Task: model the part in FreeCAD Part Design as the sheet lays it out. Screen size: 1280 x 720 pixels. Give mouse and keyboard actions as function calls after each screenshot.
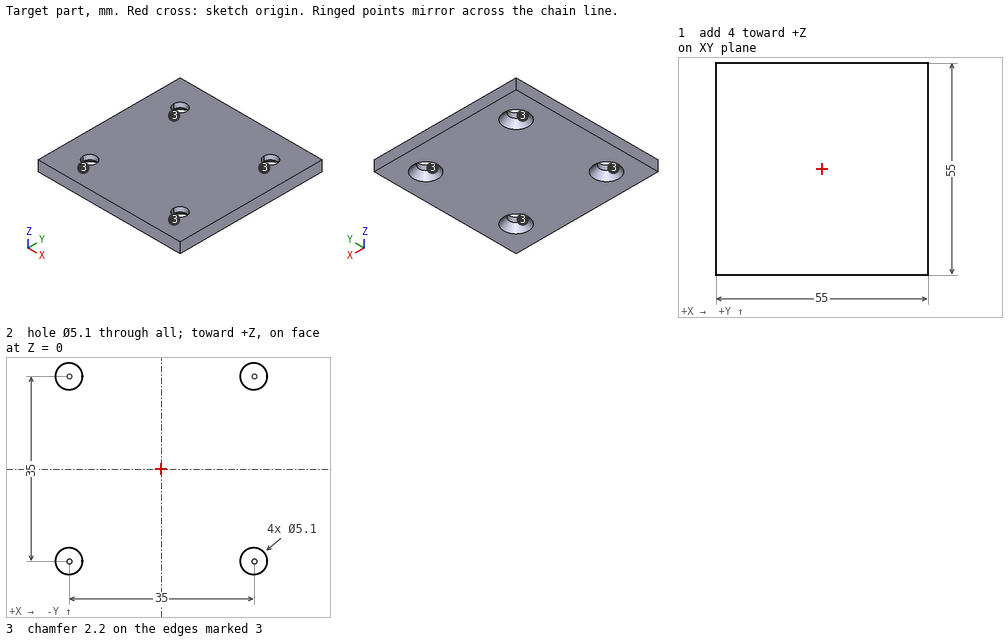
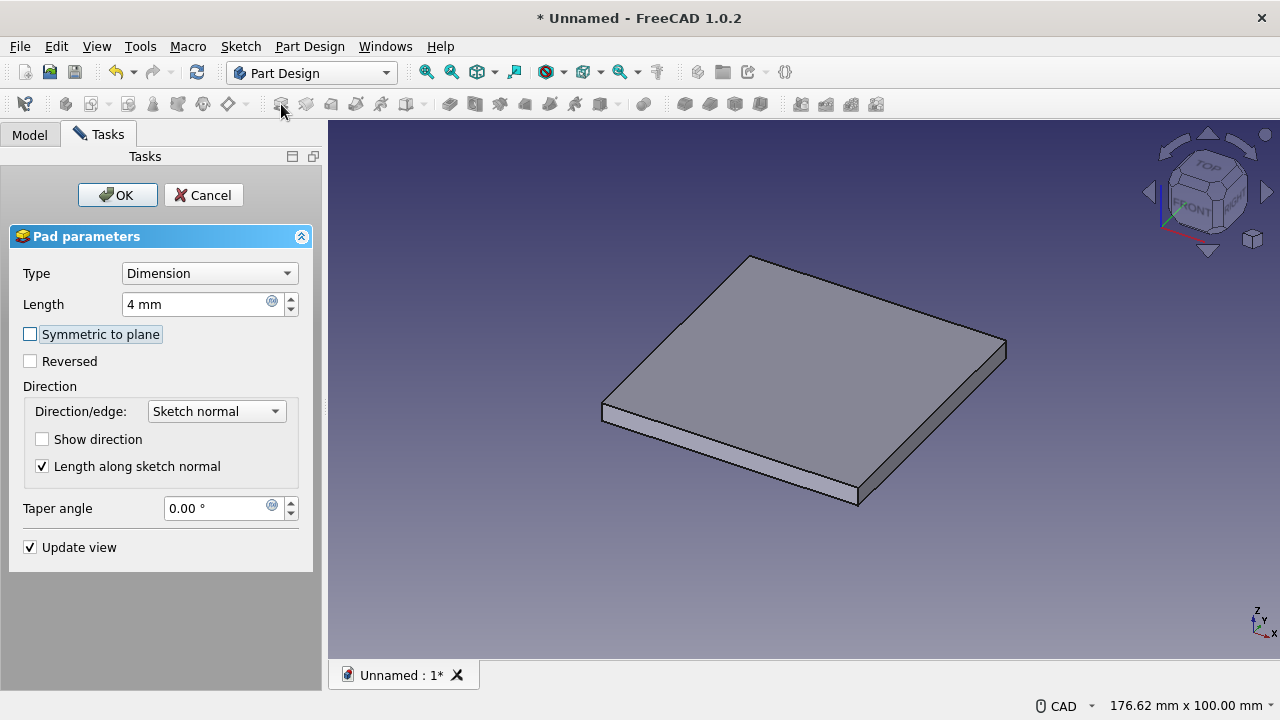
click(118, 195)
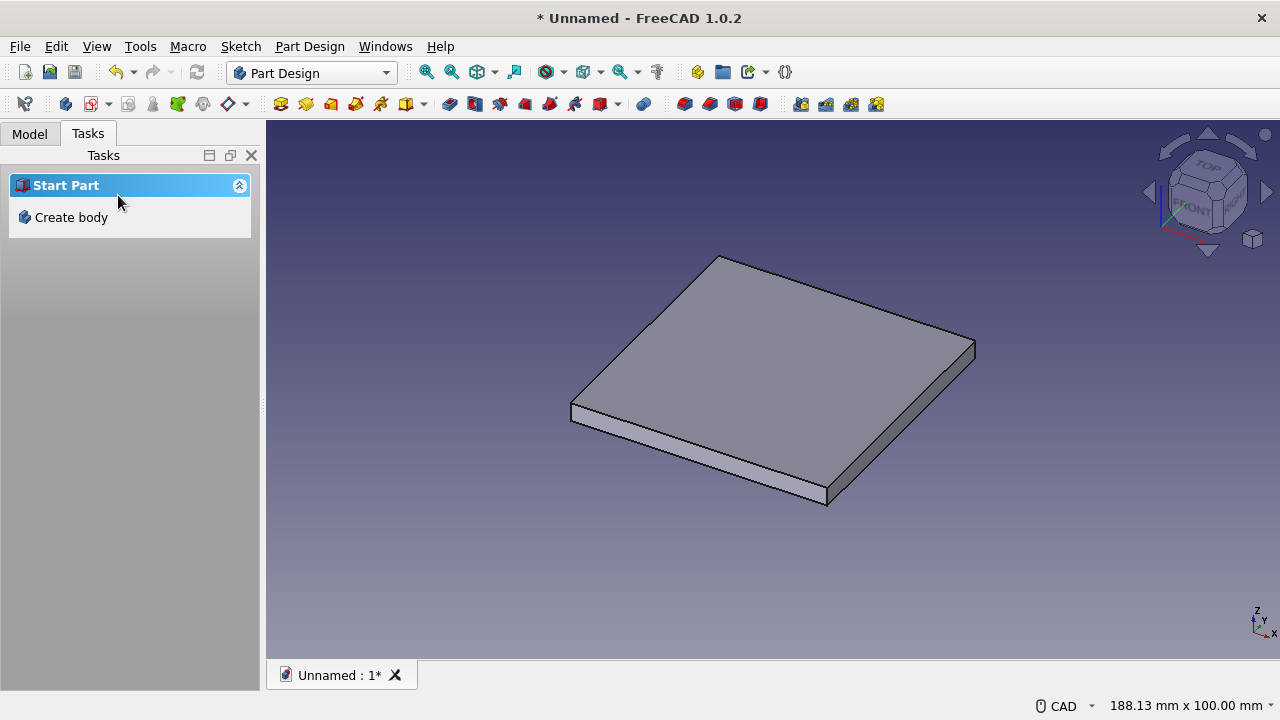
key(5)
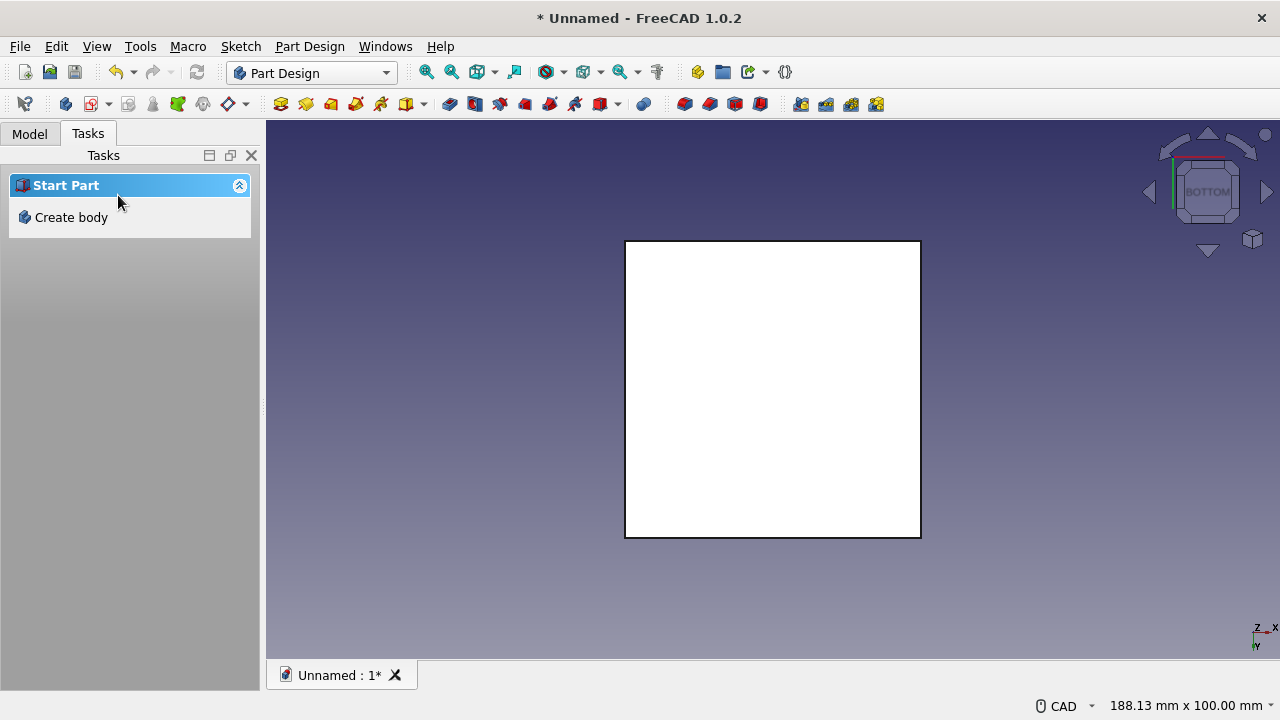
click(773, 388)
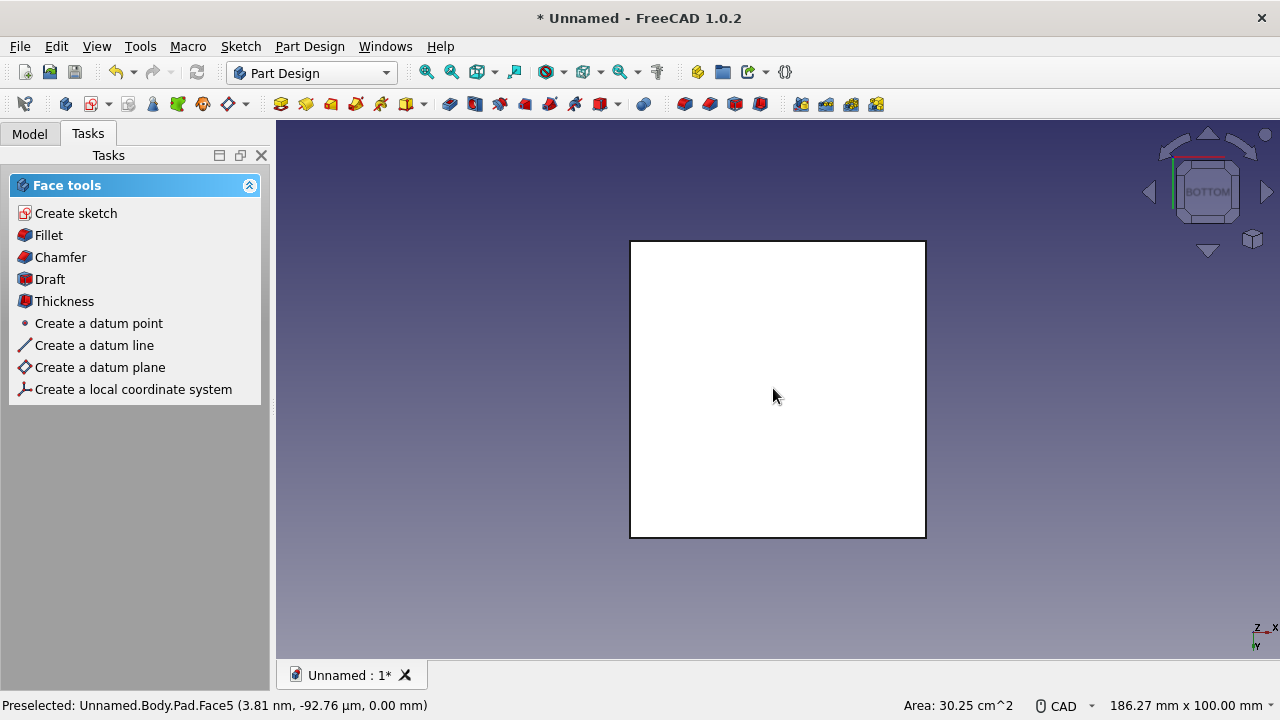
click(90, 104)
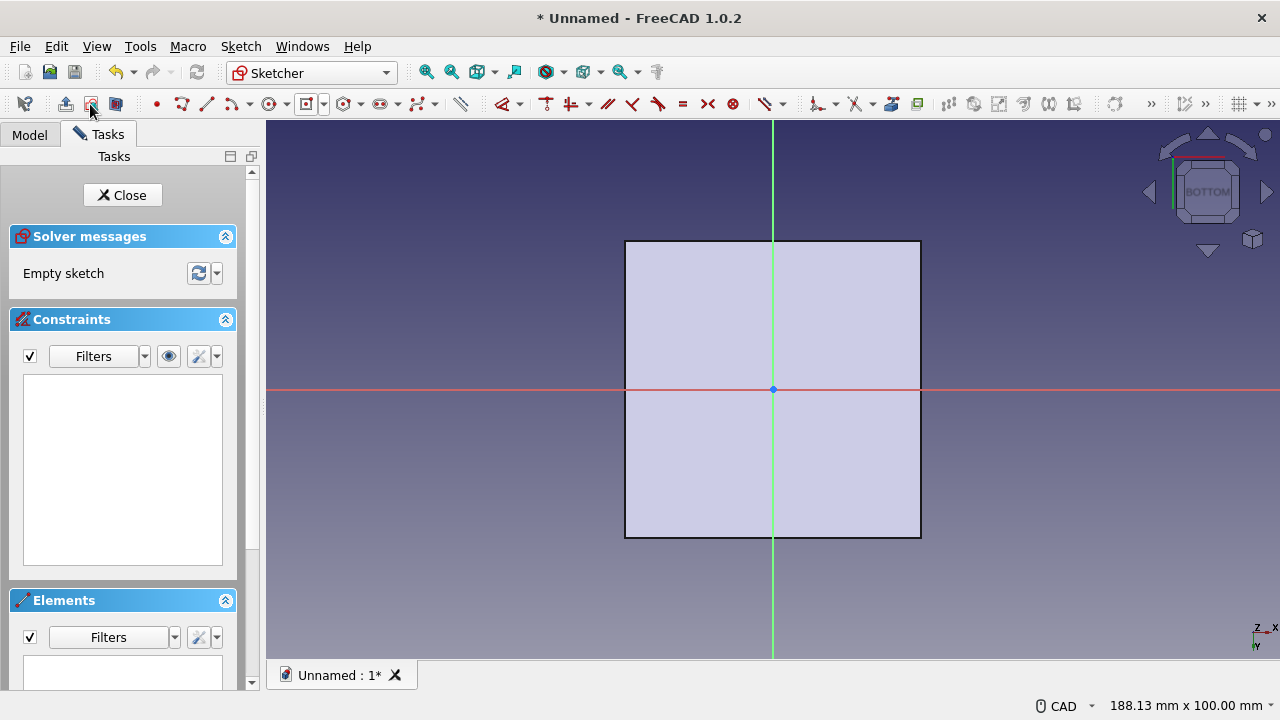
scroll(912, 390, up, 2)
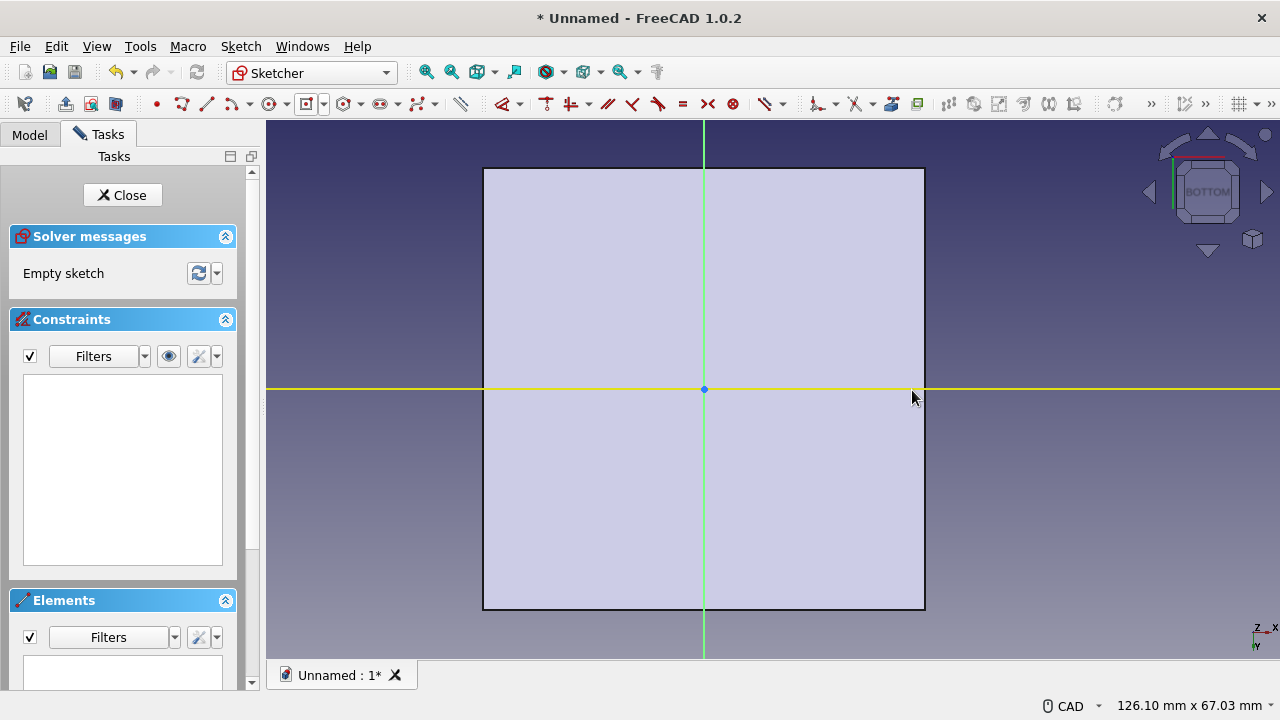
click(268, 104)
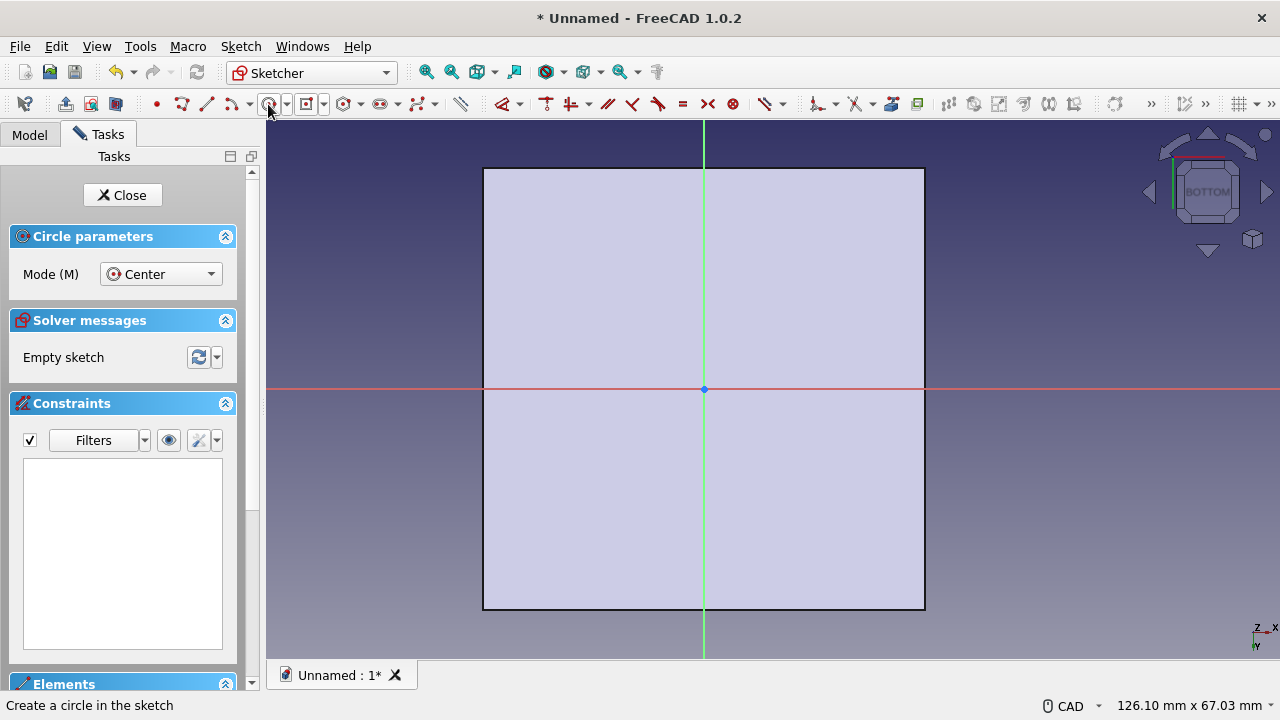
click(845, 530)
move(860, 515)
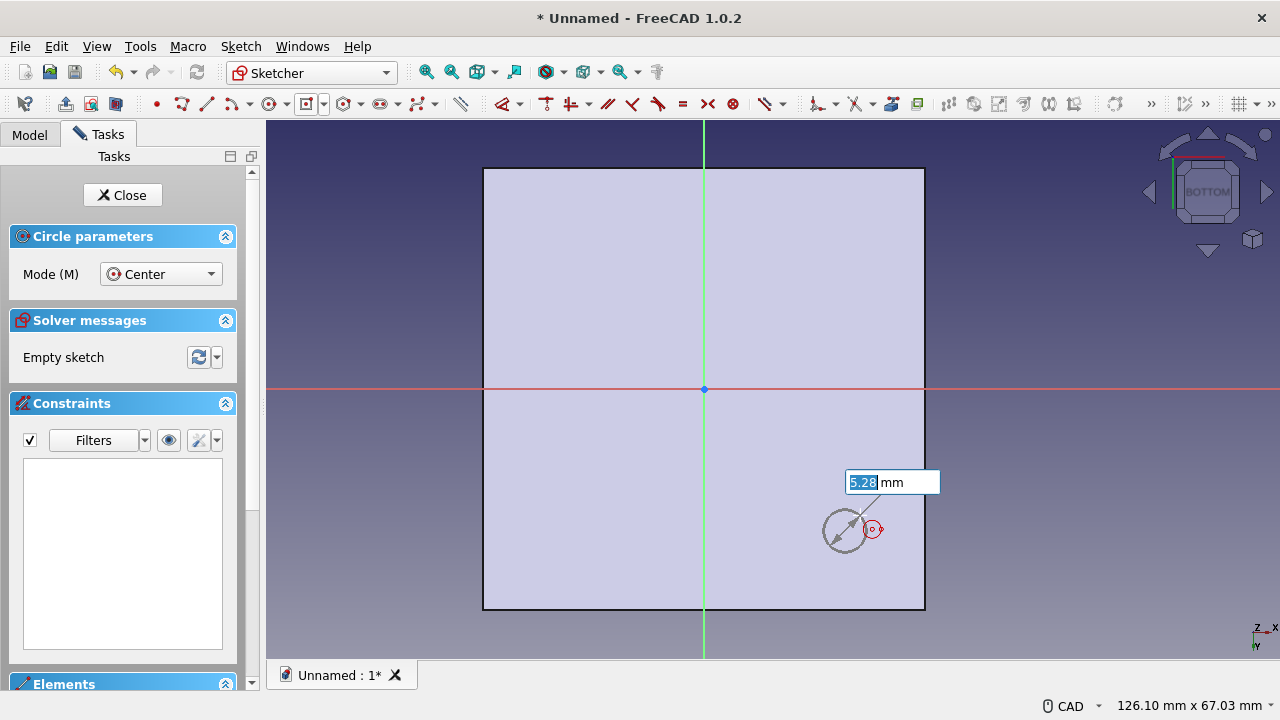
text(5.1)
key(Return)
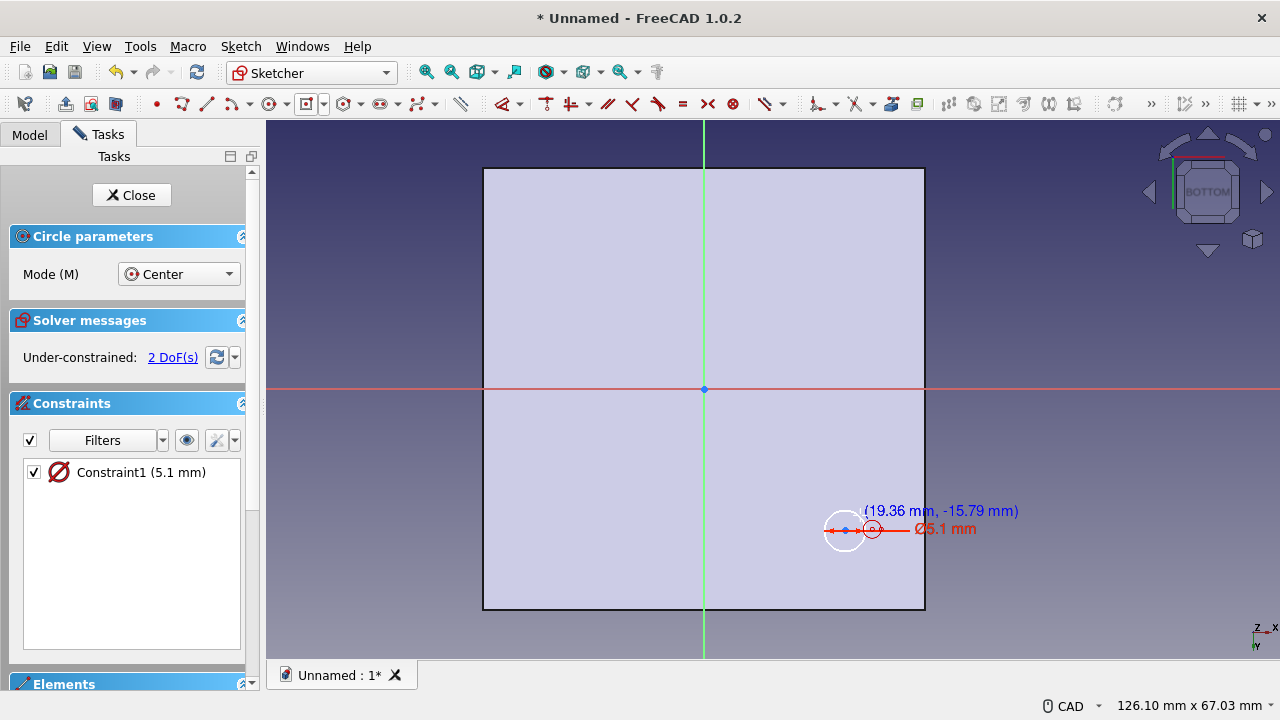
click(564, 530)
move(578, 515)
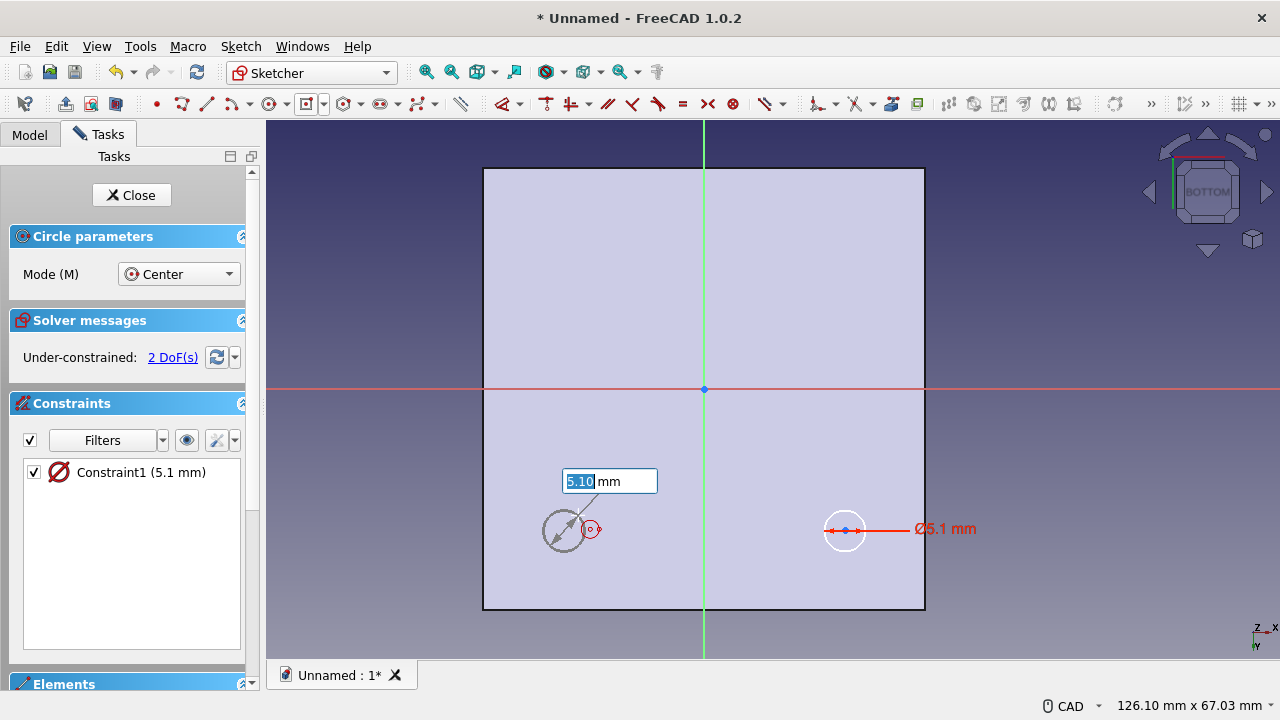
text(5.1)
key(Return)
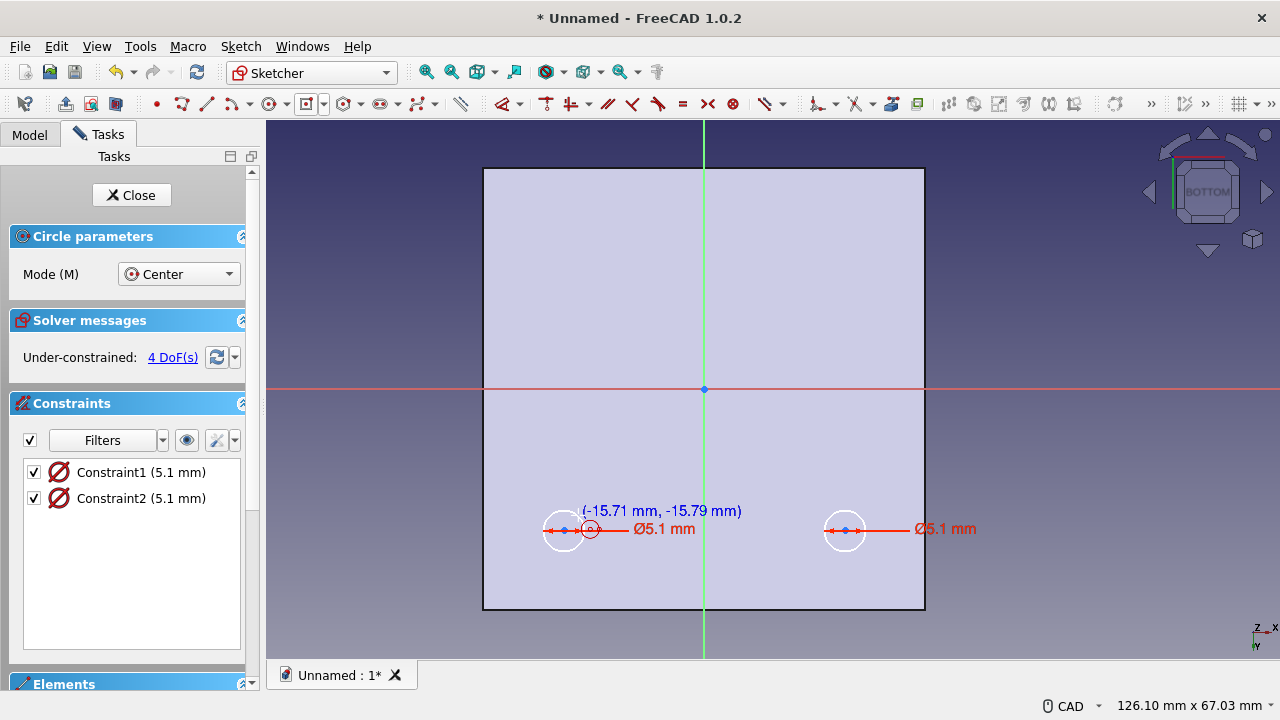
click(564, 248)
move(578, 234)